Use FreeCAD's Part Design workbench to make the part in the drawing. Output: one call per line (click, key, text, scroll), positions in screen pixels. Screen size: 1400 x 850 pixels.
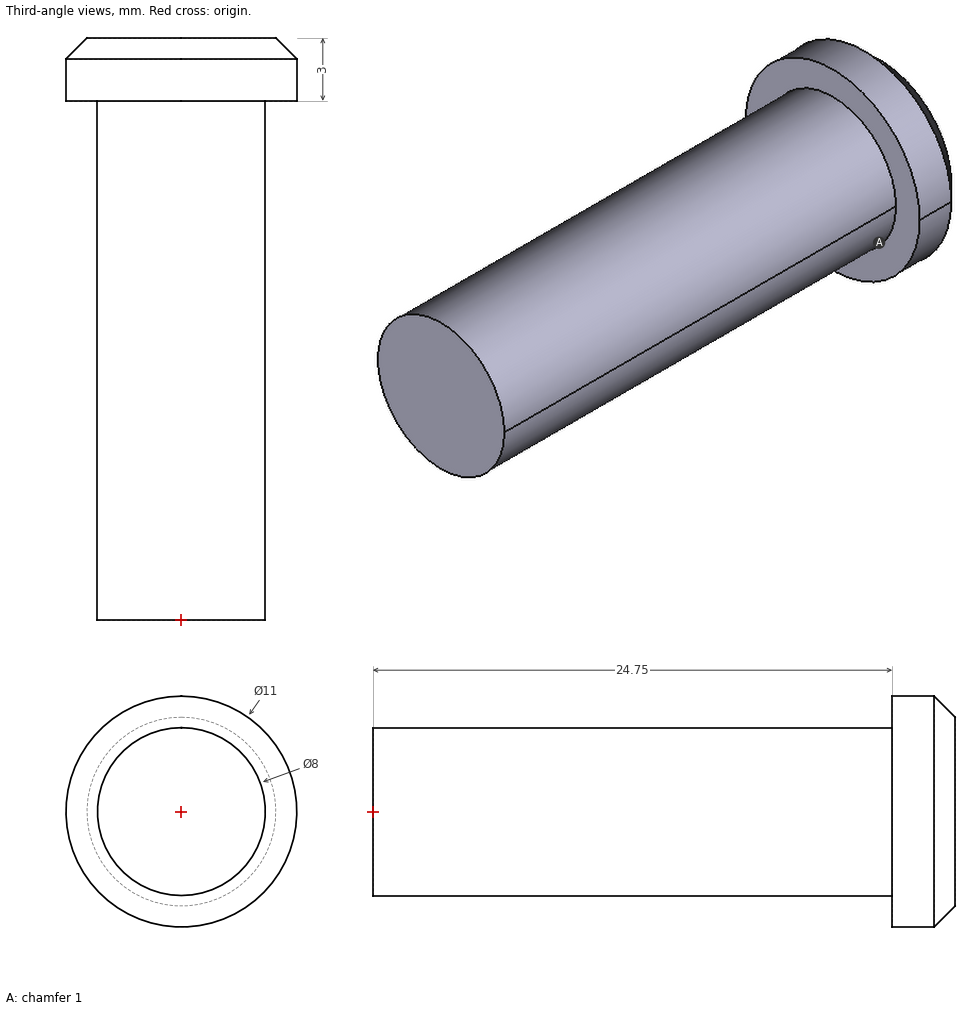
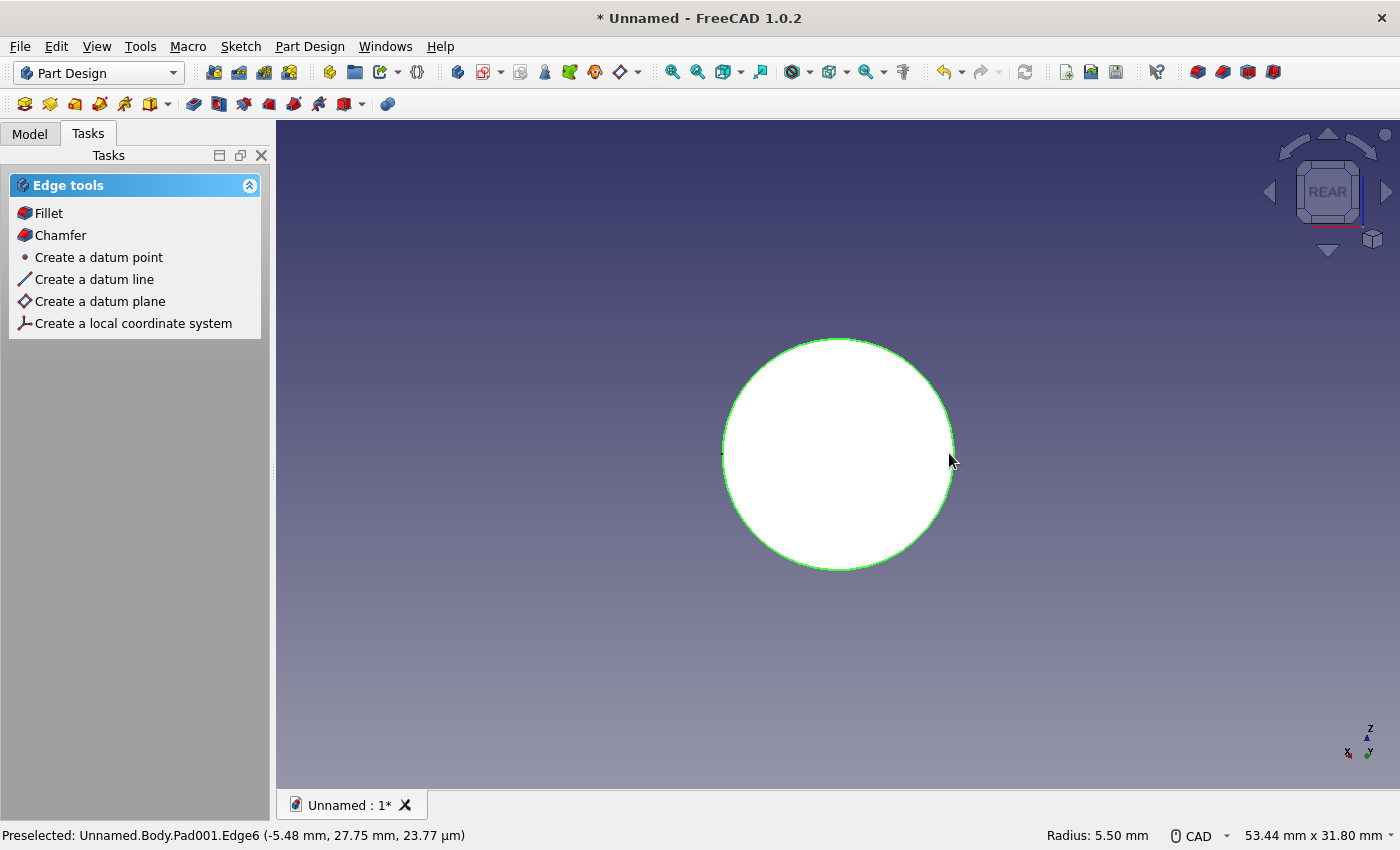
click(1223, 72)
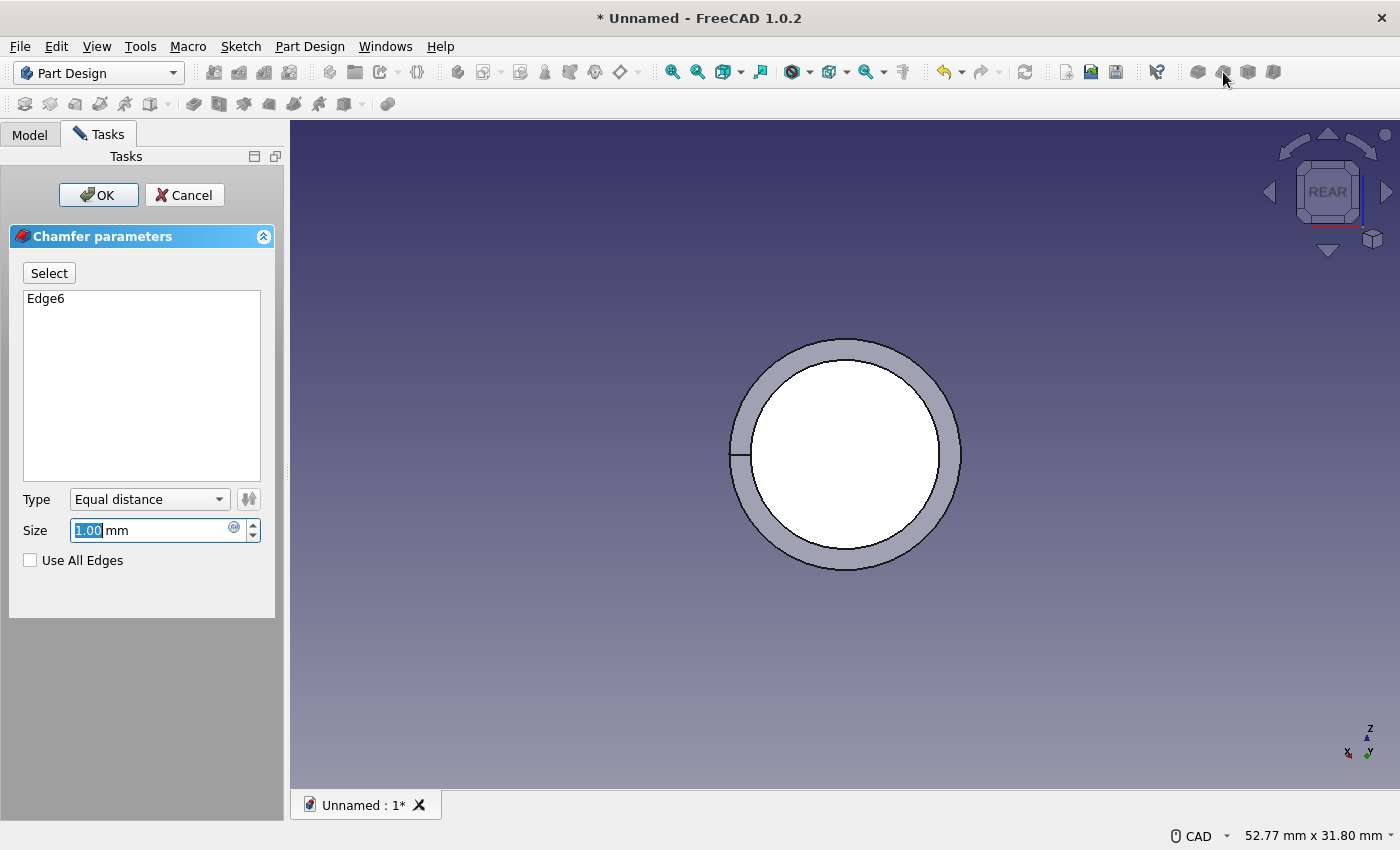
text(1)
key(Tab)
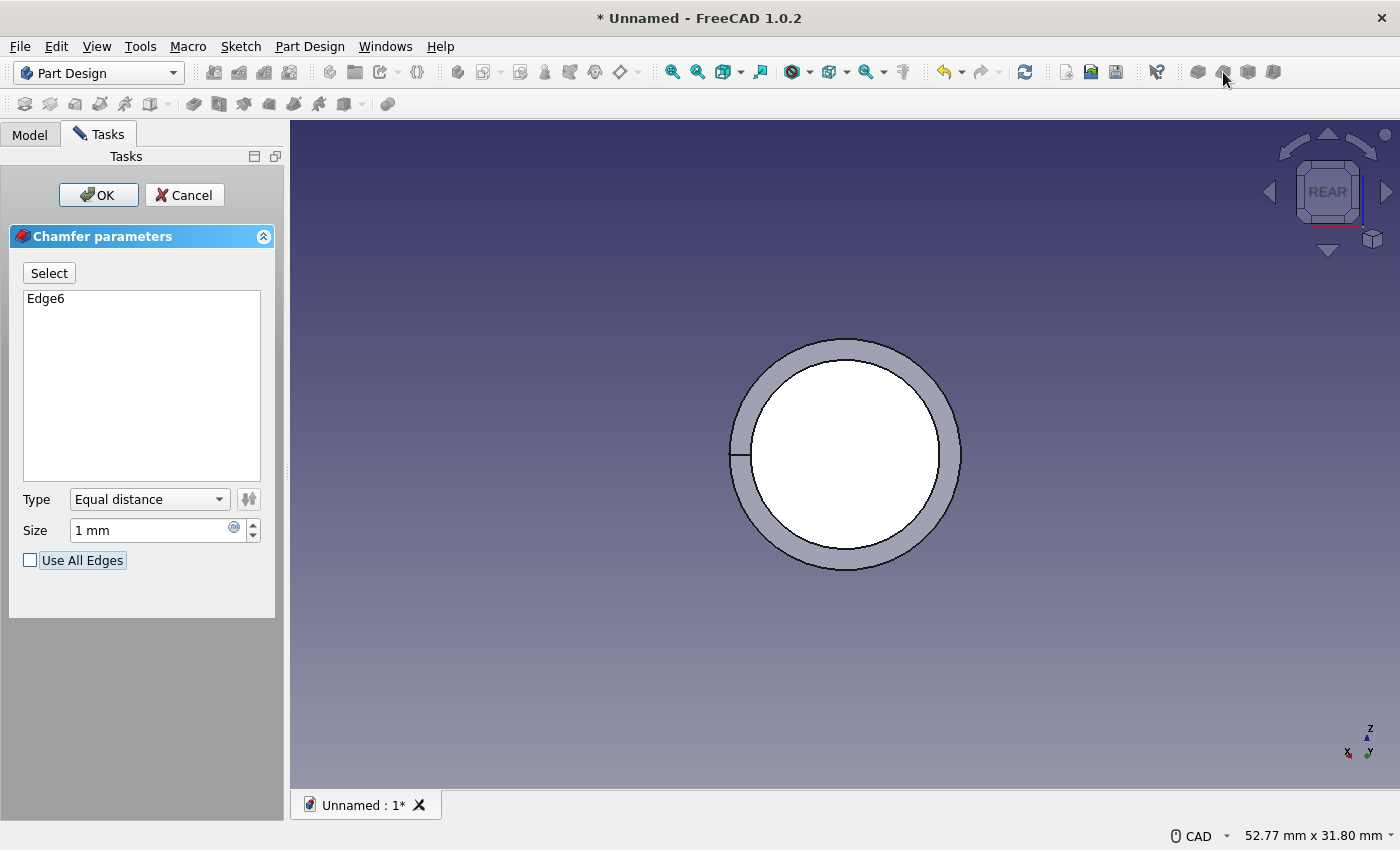
click(99, 195)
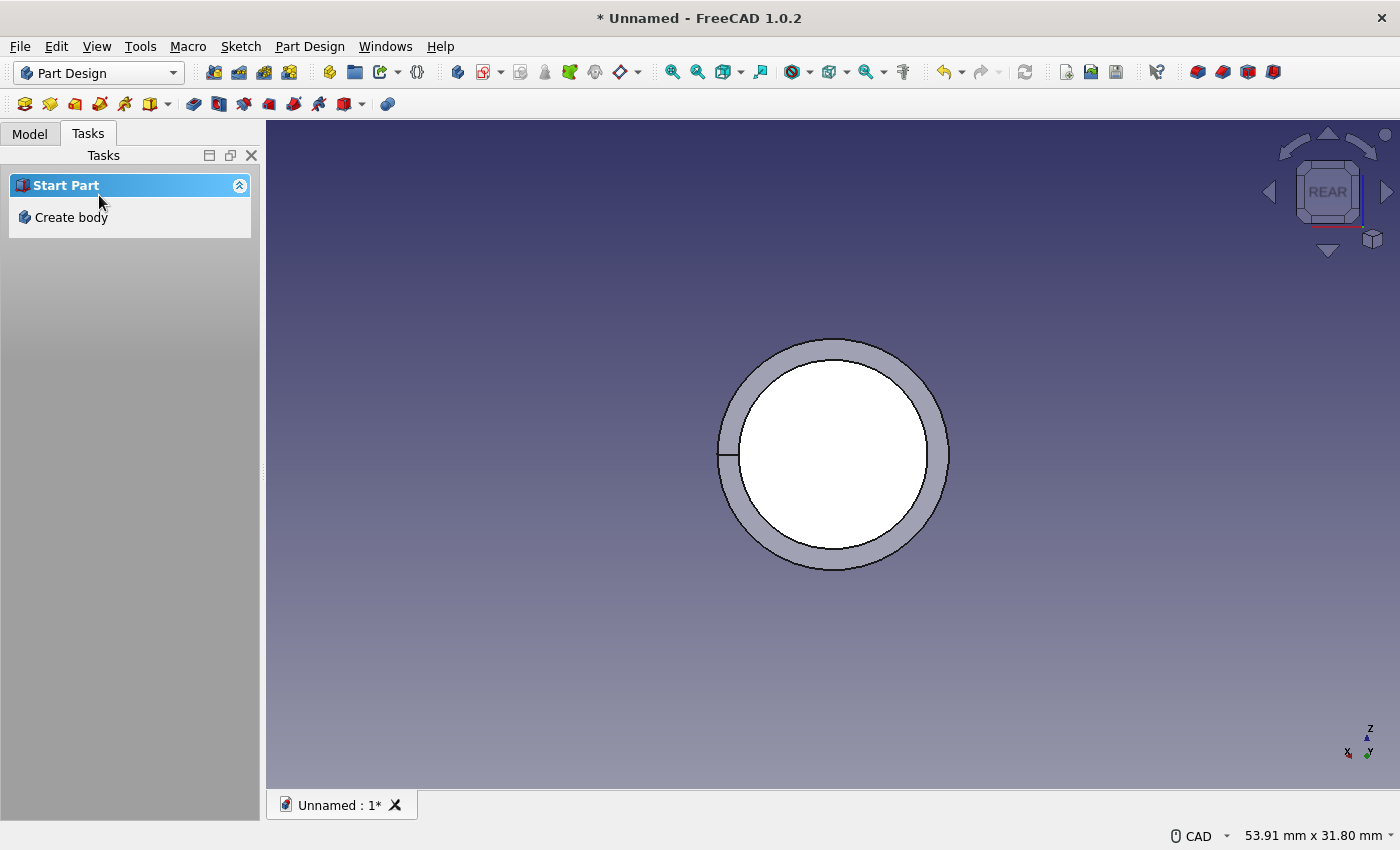
key(0)